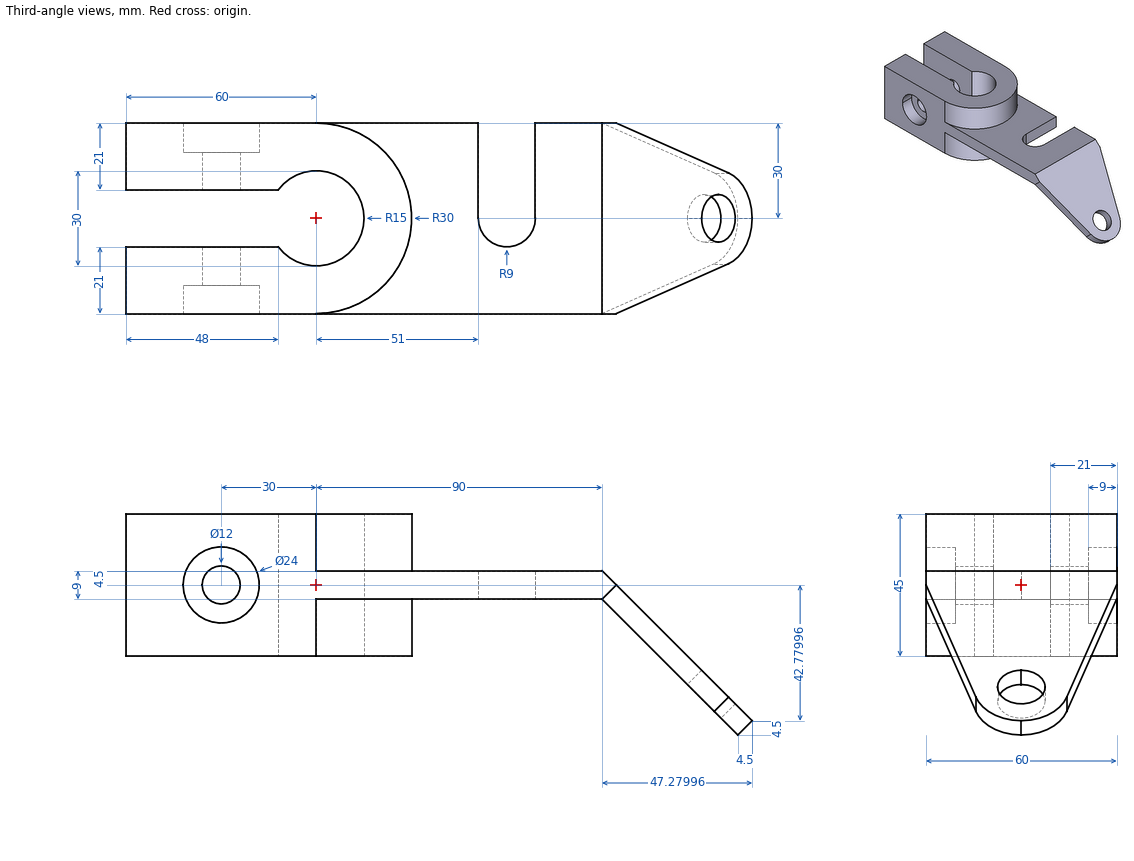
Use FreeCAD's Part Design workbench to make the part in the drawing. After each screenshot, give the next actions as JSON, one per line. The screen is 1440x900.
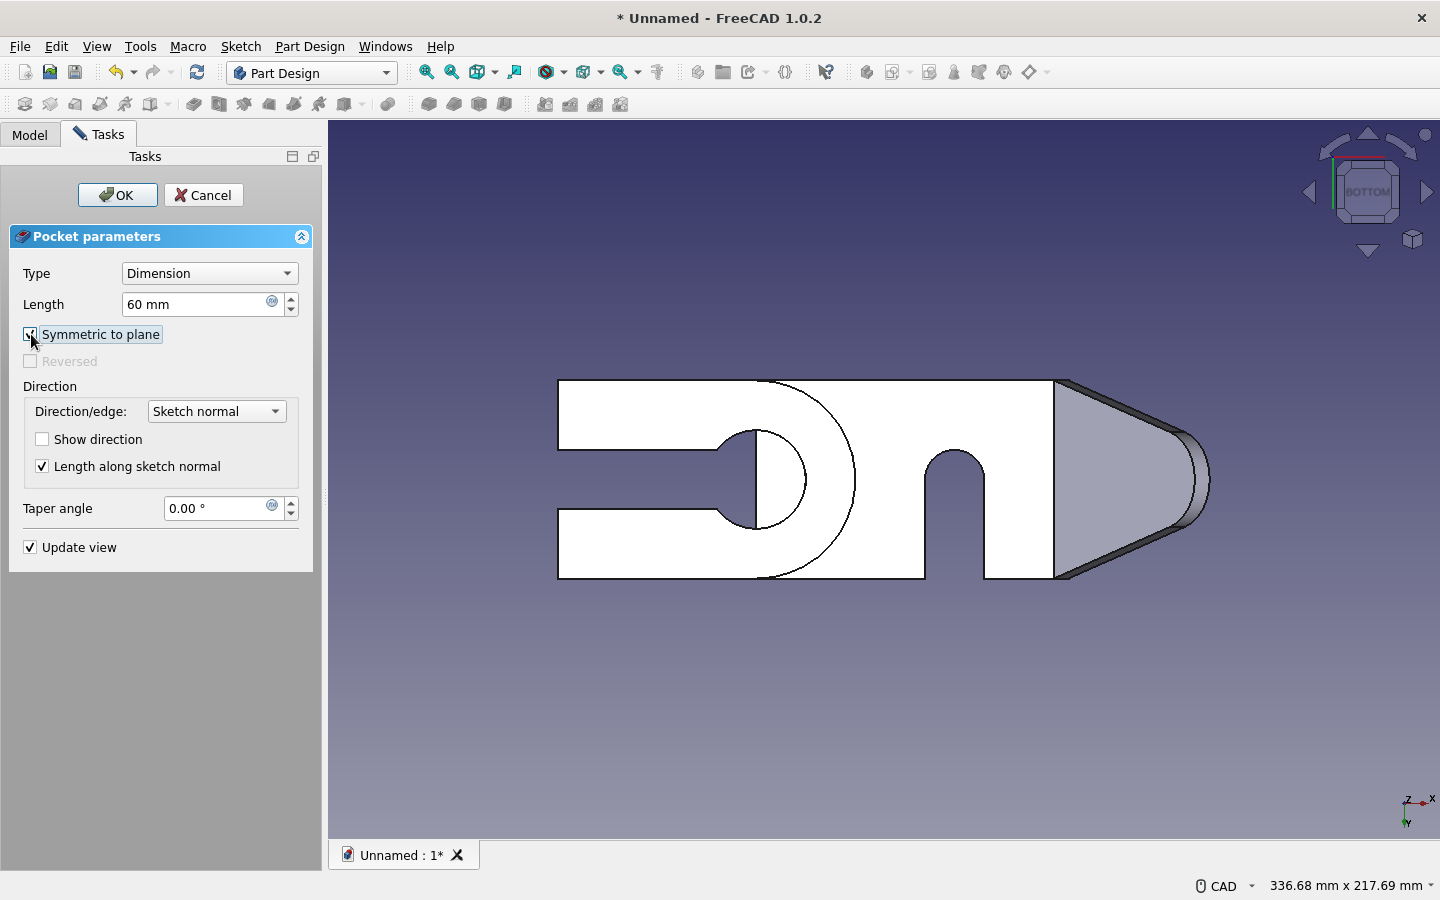
{"action": "left_click", "coordinate": [118, 195]}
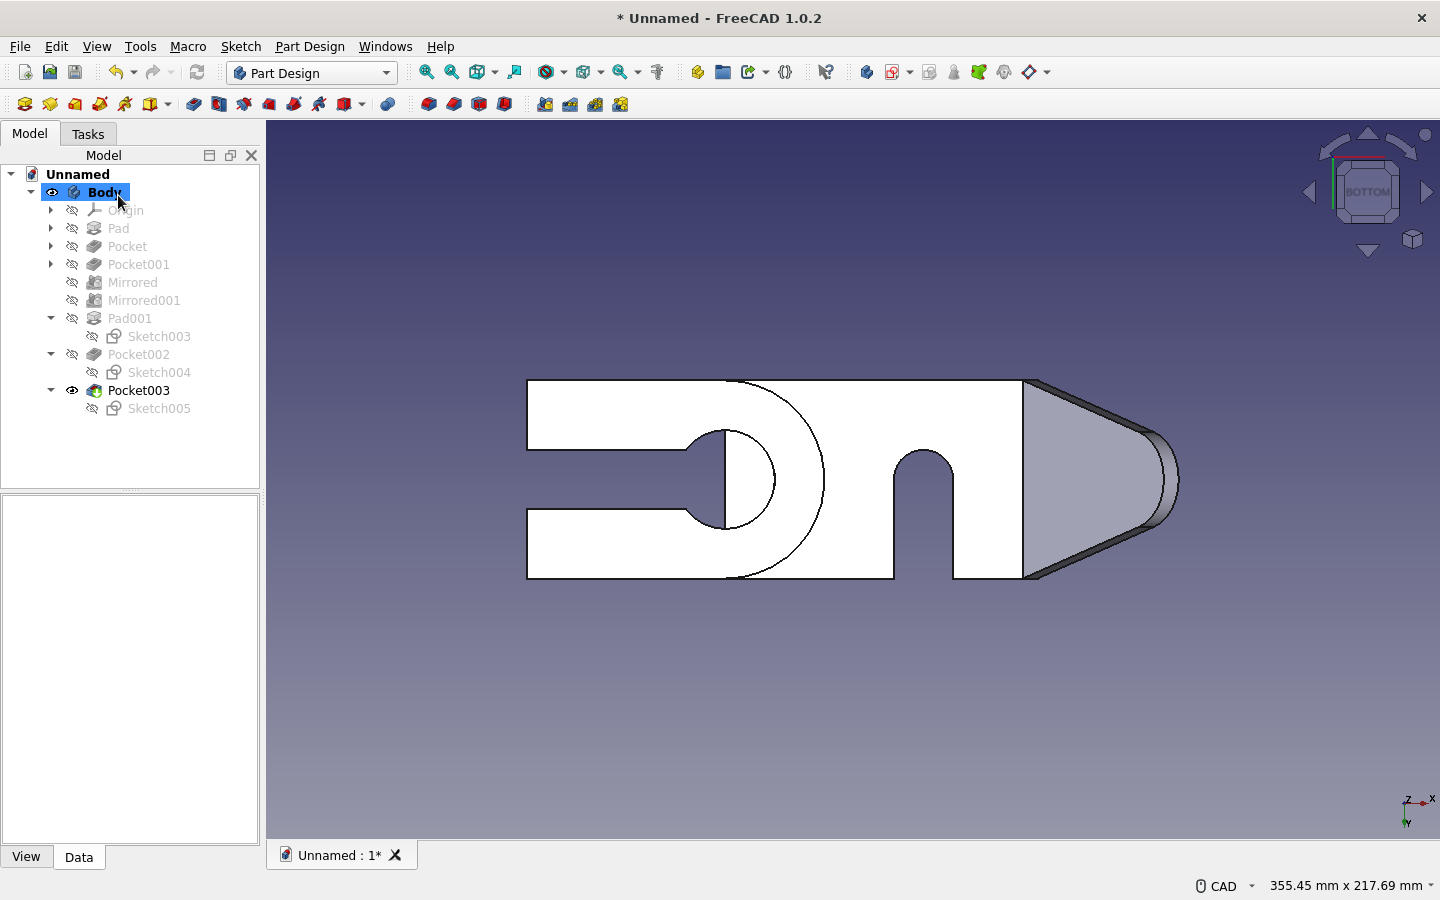
{"action": "left_click", "coordinate": [1073, 479]}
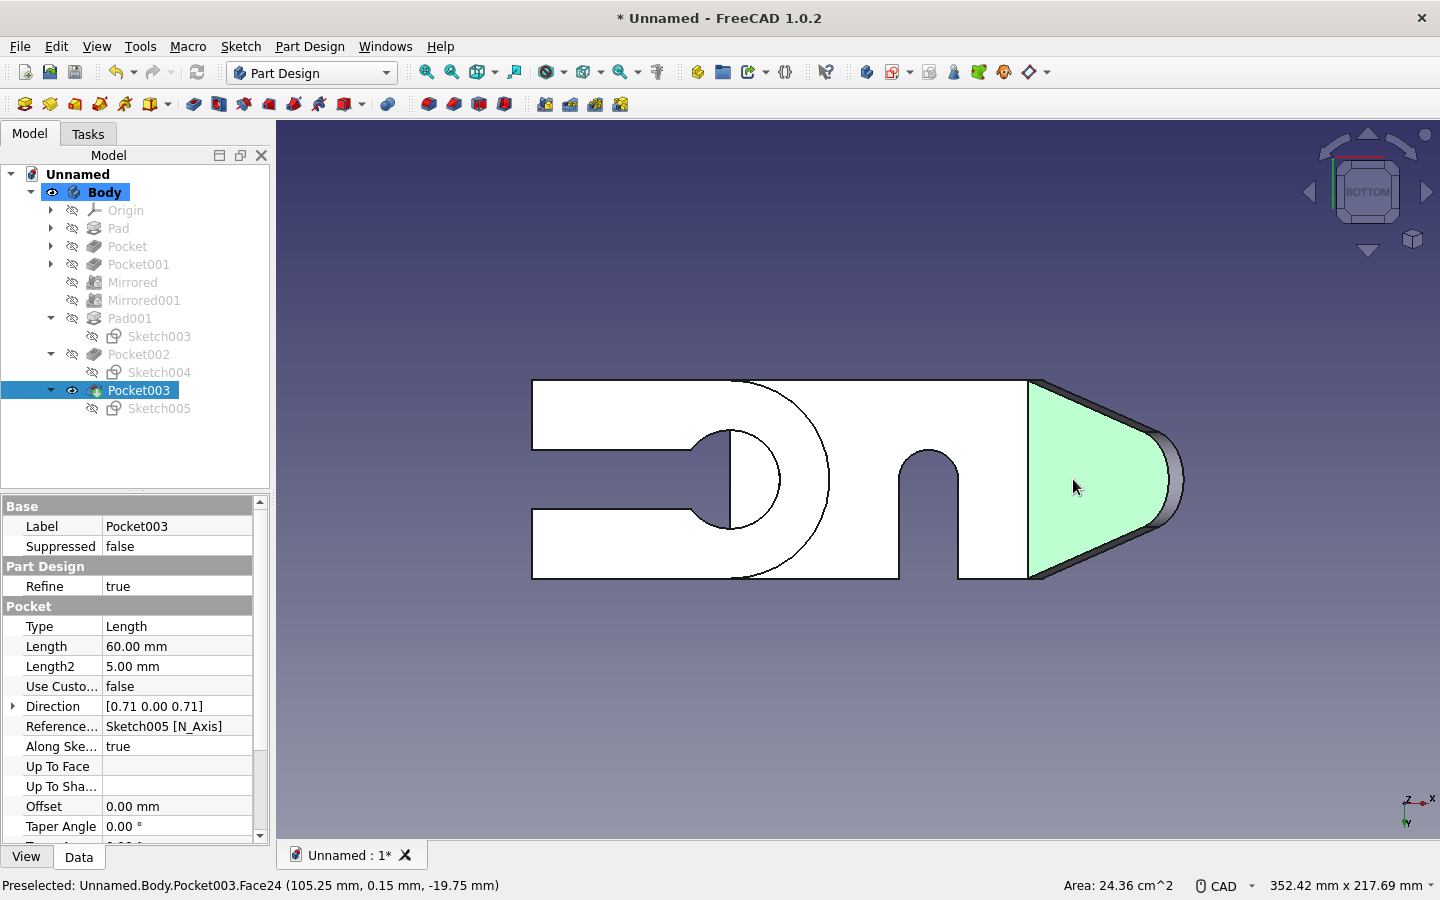
{"action": "left_click", "coordinate": [892, 72]}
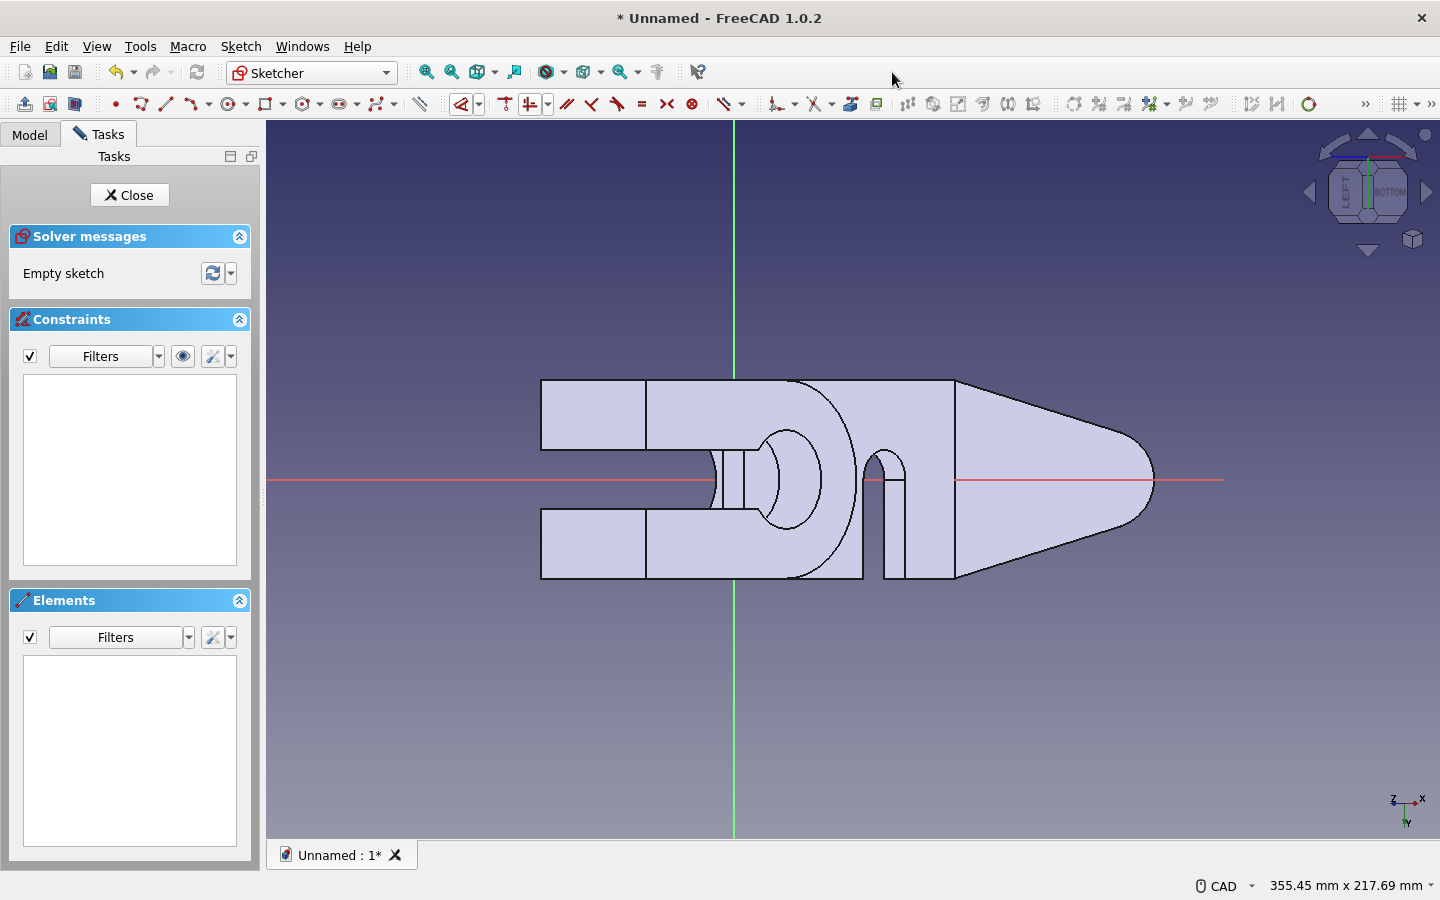
{"action": "left_click", "coordinate": [75, 104]}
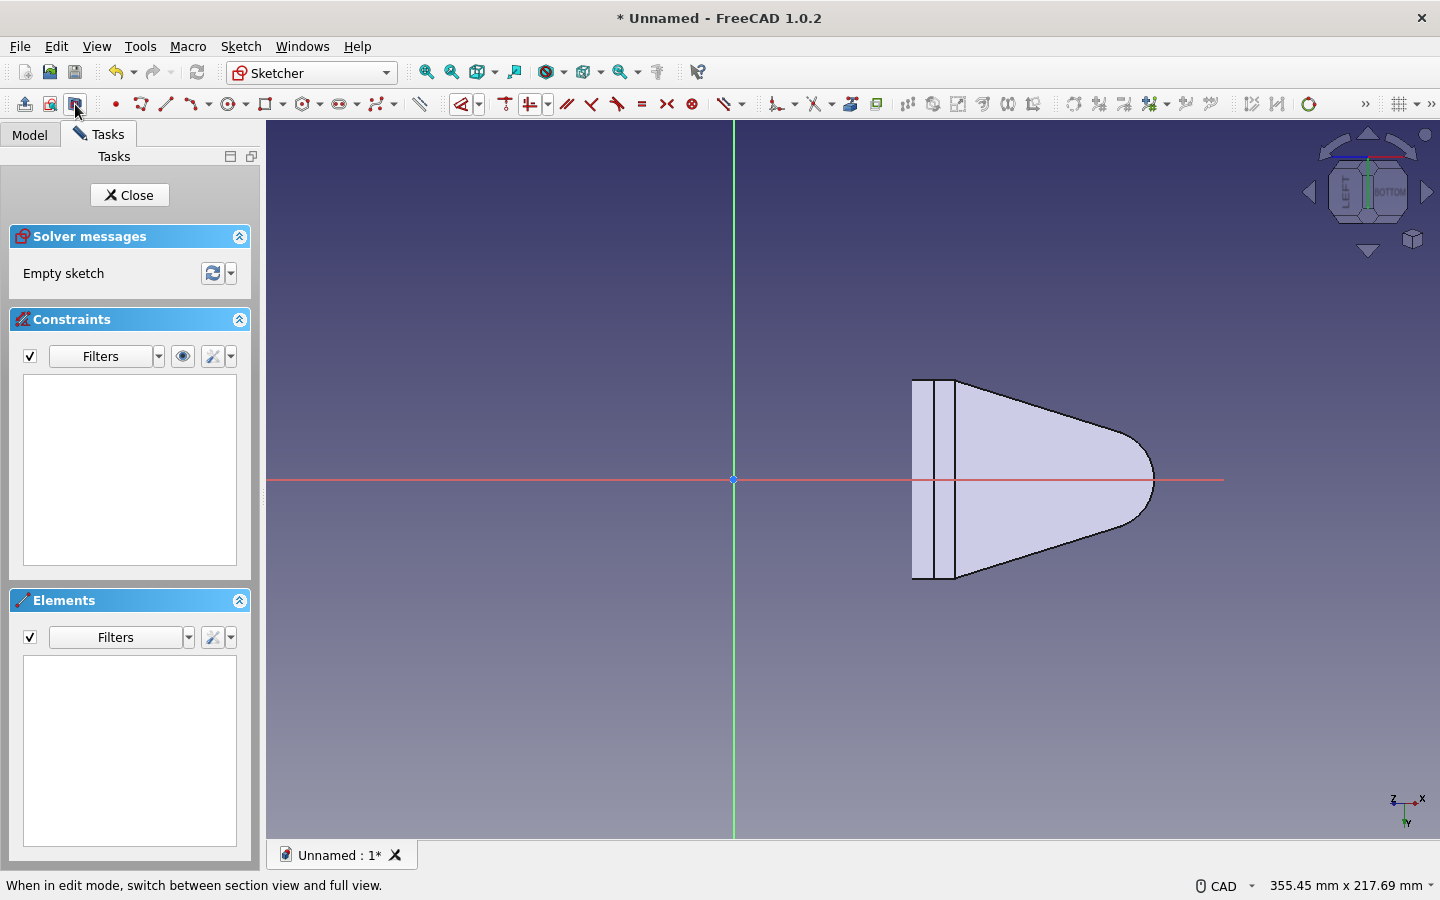
{"action": "scroll", "coordinate": [1145, 480], "scroll_direction": "up", "scroll_amount": 11}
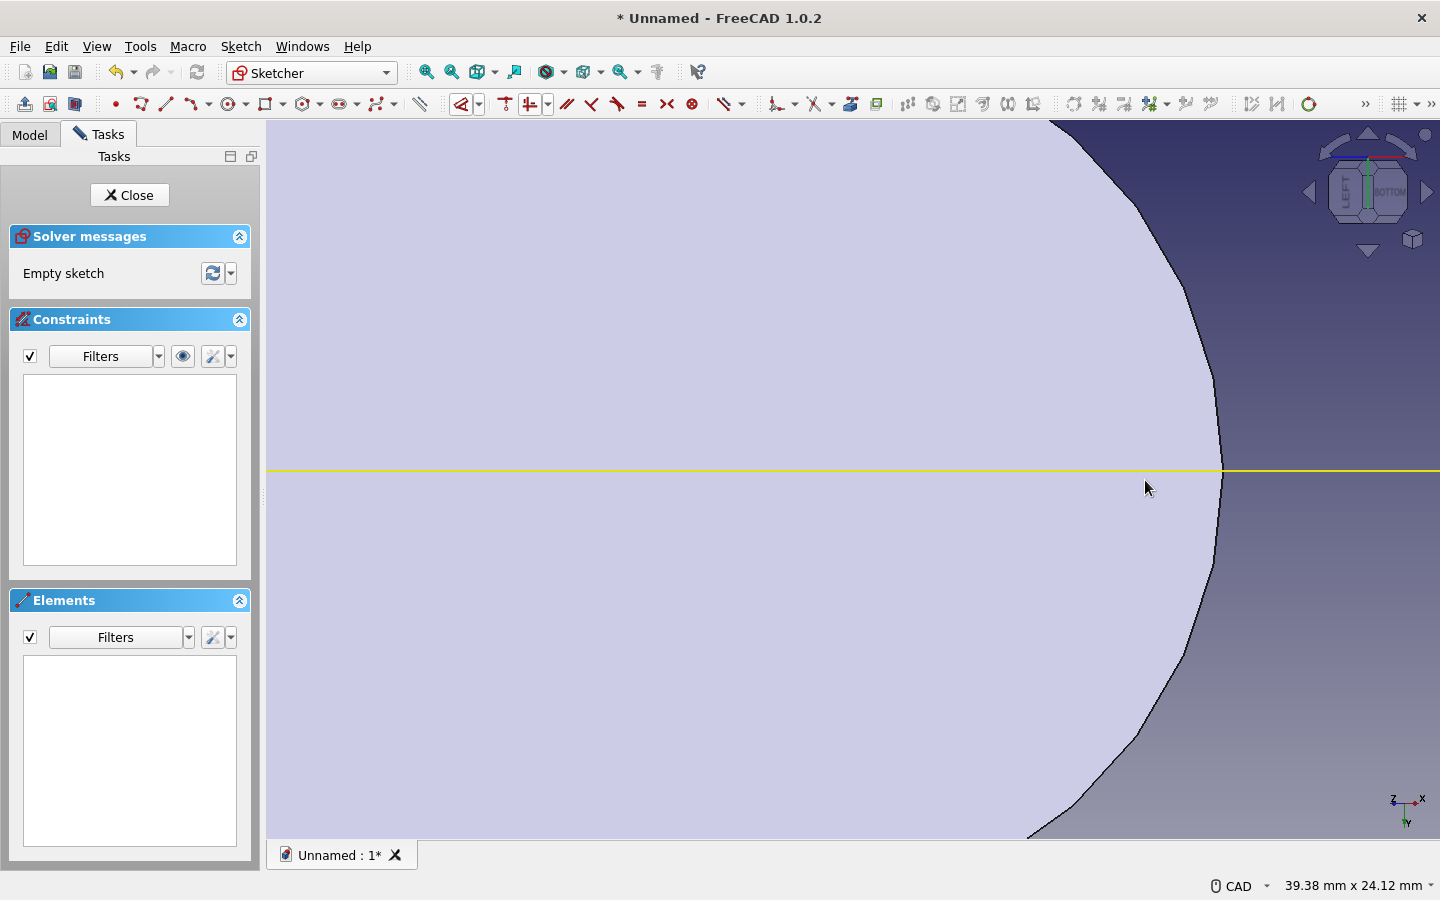
{"action": "left_click", "coordinate": [228, 104]}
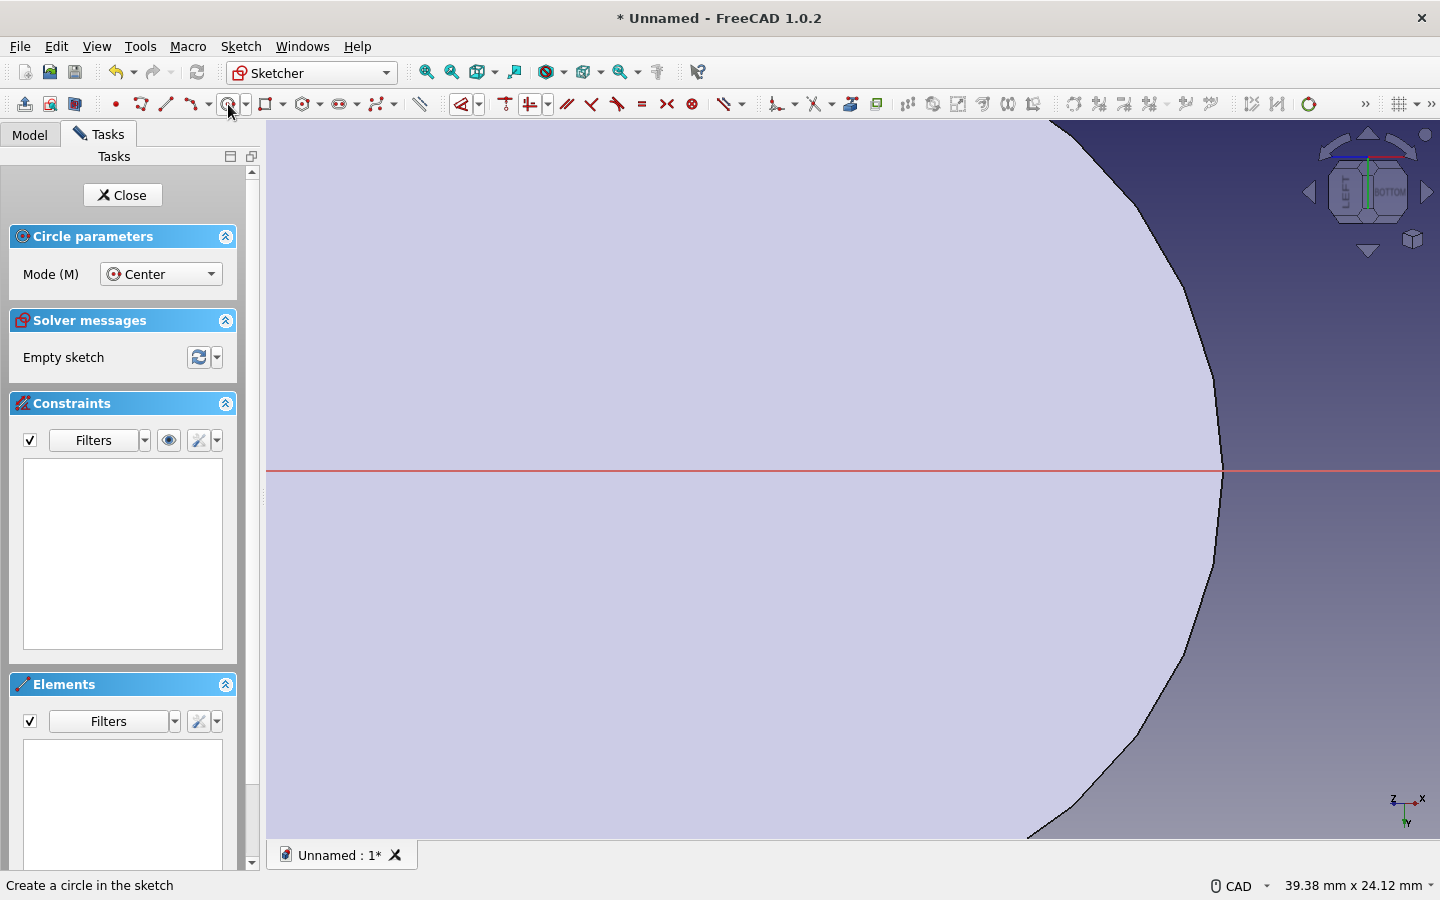
{"action": "left_click", "coordinate": [776, 471]}
{"action": "left_click", "coordinate": [934, 313]}
{"action": "key", "text": "Escape"}